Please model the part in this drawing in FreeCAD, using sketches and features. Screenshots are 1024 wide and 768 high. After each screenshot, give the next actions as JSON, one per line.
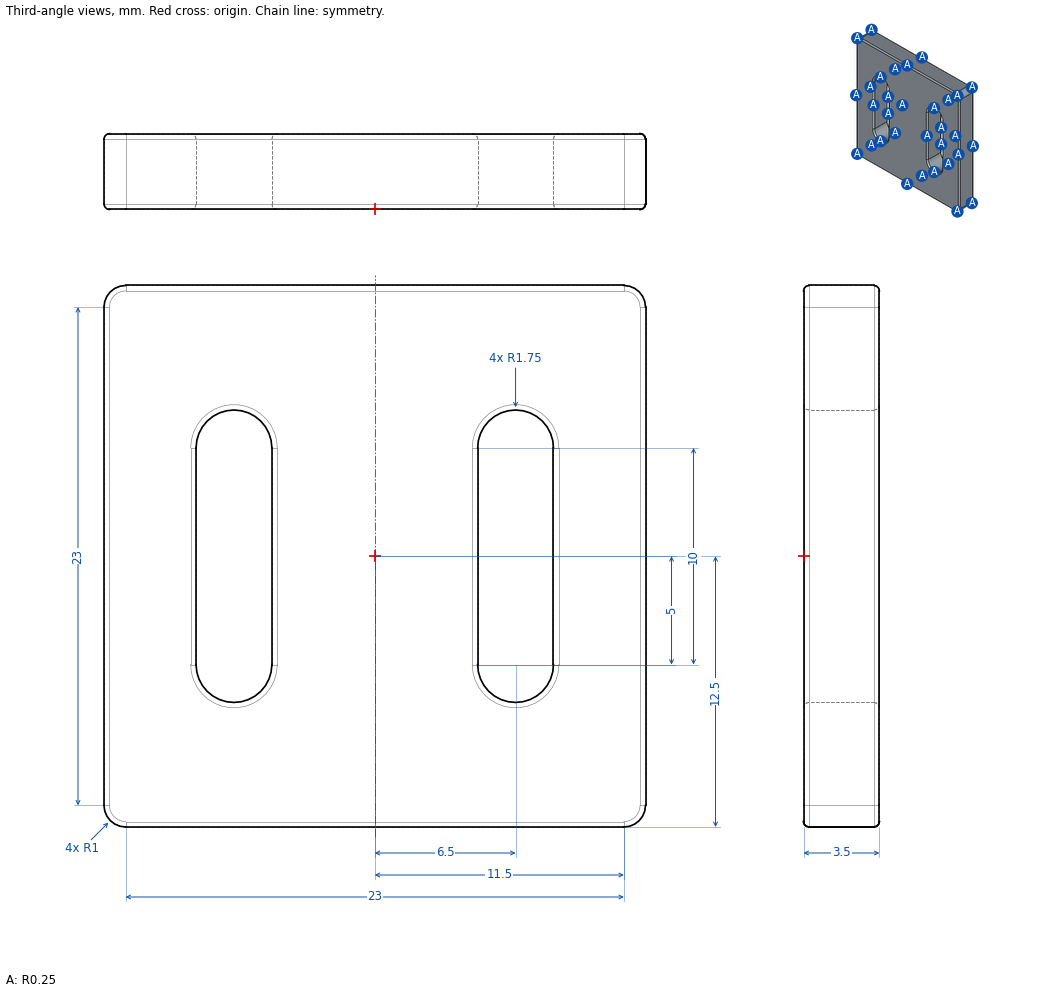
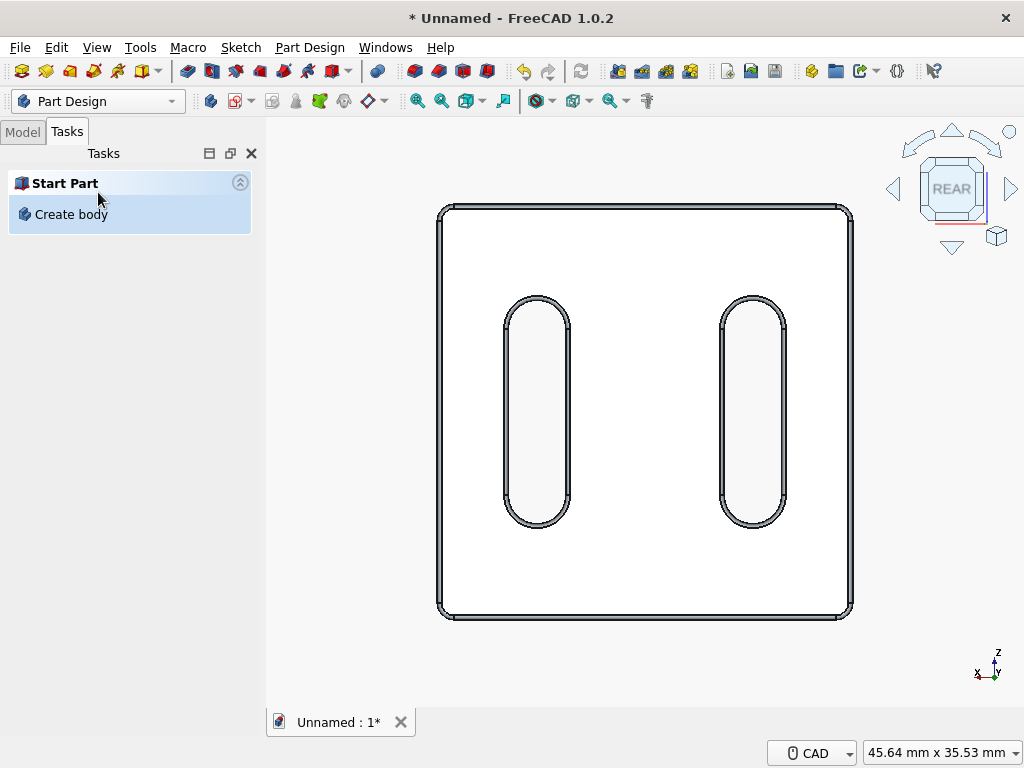
{"action": "key", "text": "0"}